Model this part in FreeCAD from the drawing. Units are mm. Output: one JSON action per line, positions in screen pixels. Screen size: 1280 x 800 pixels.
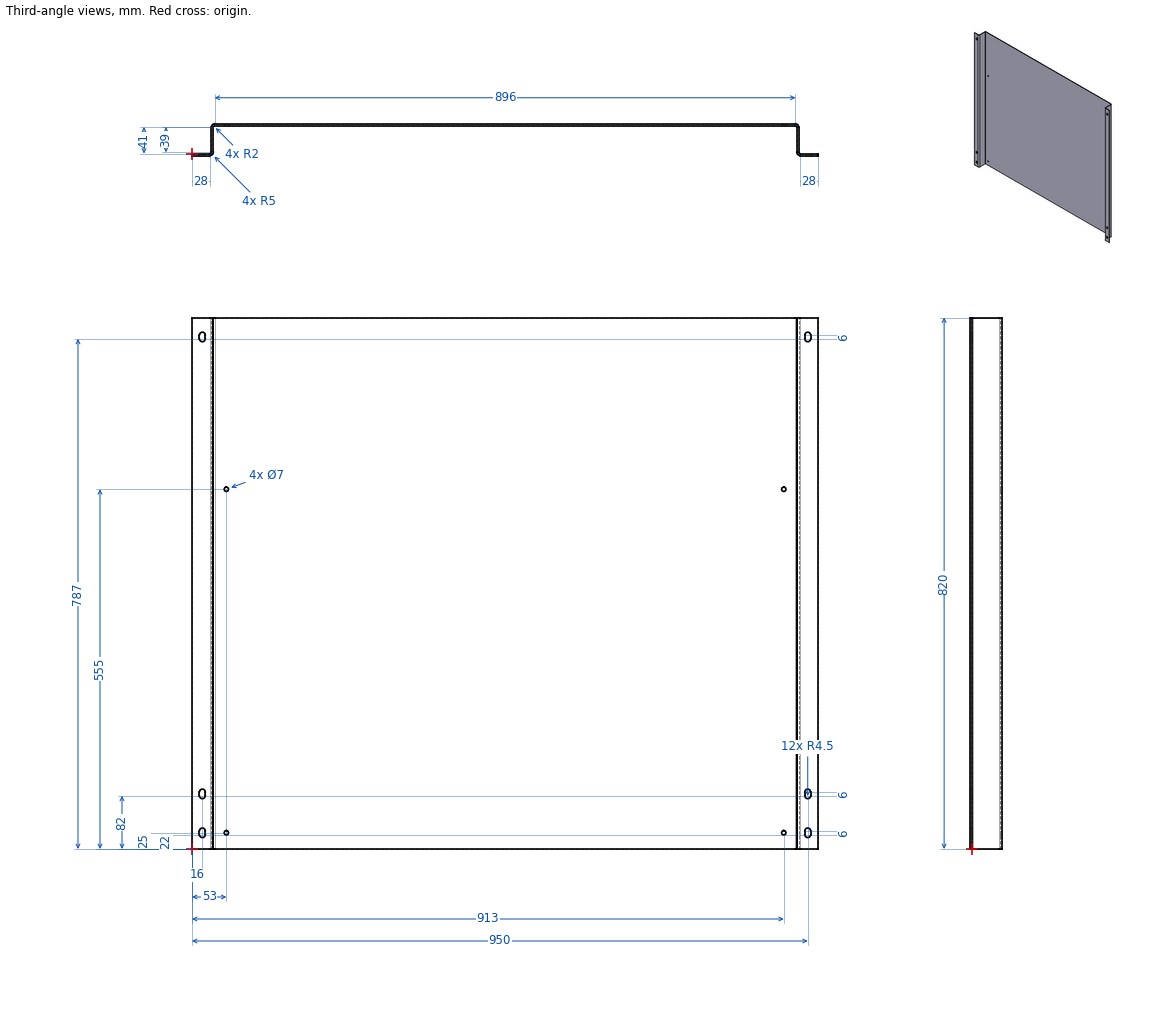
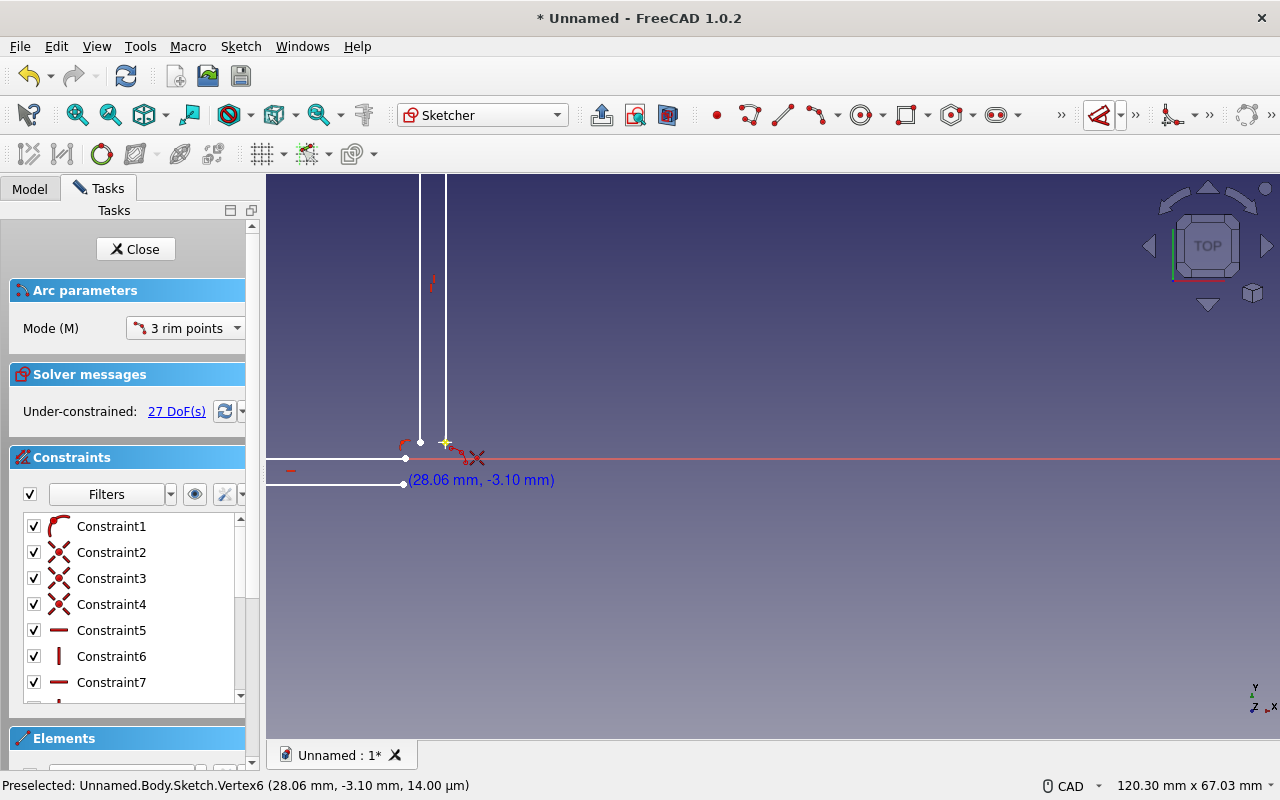
{"action": "left_click", "coordinate": [446, 443]}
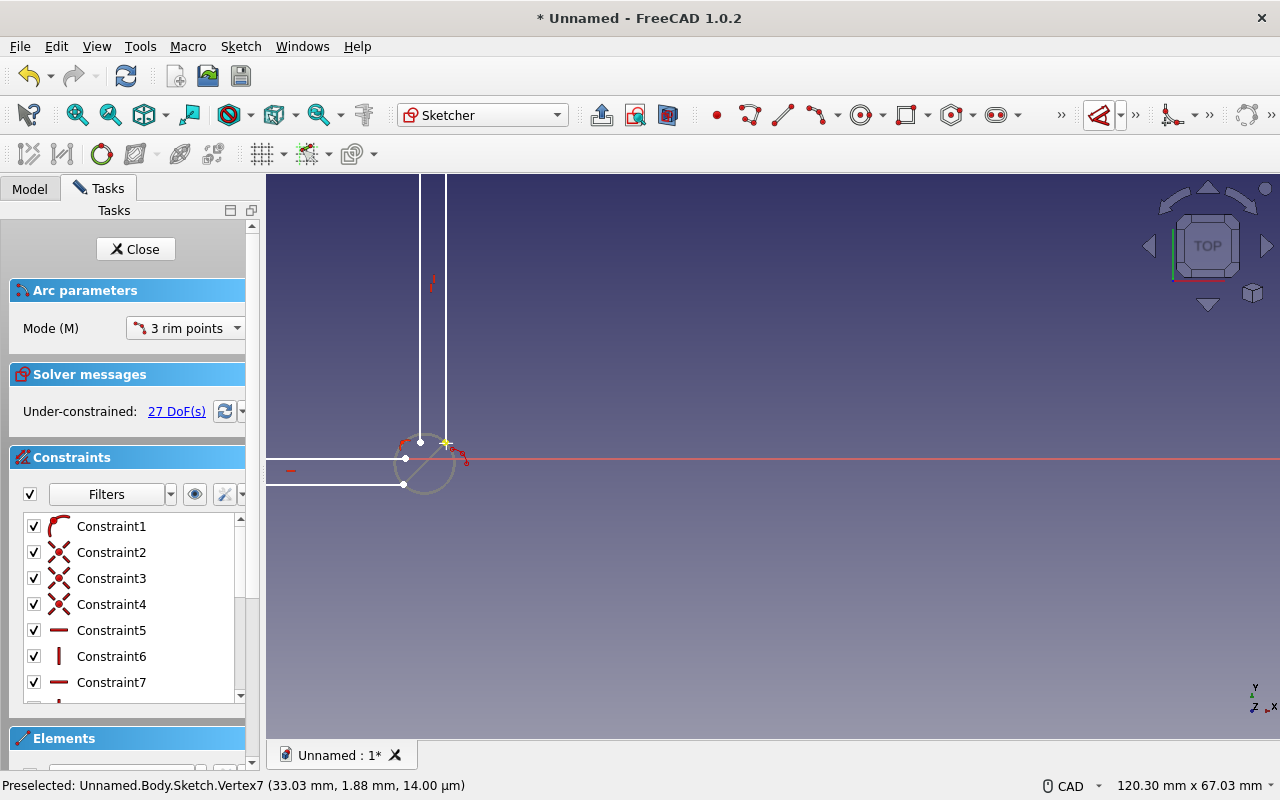
{"action": "scroll", "coordinate": [433, 471], "scroll_direction": "up", "scroll_amount": 2}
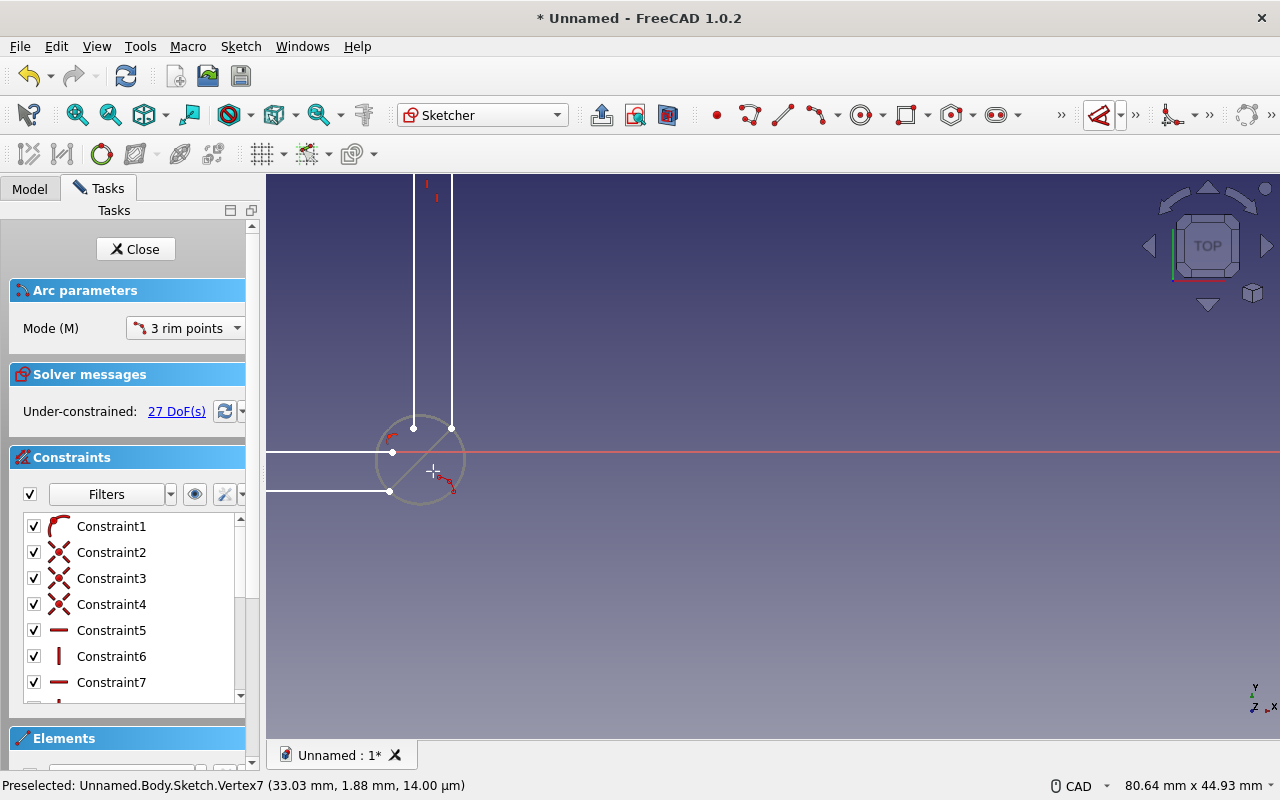
{"action": "left_click", "coordinate": [433, 471]}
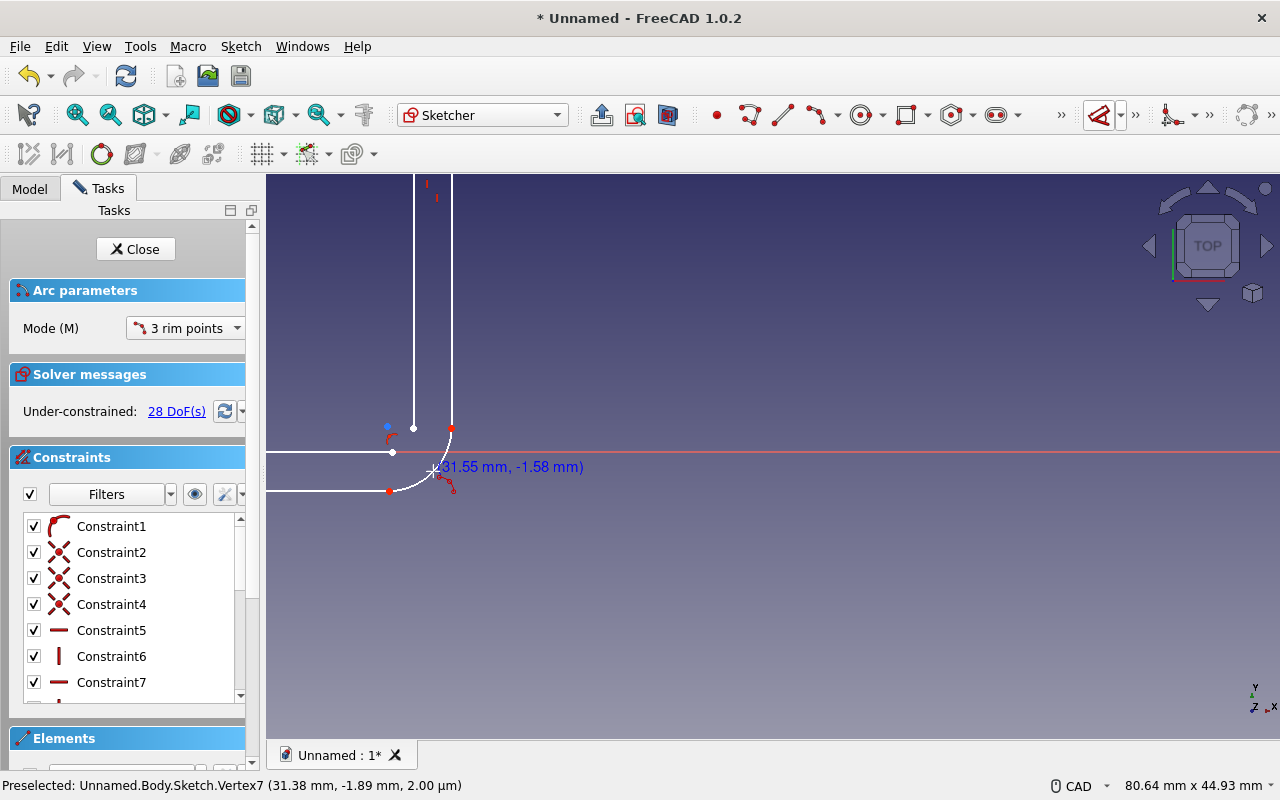
{"action": "scroll", "coordinate": [421, 471], "scroll_direction": "down", "scroll_amount": 15}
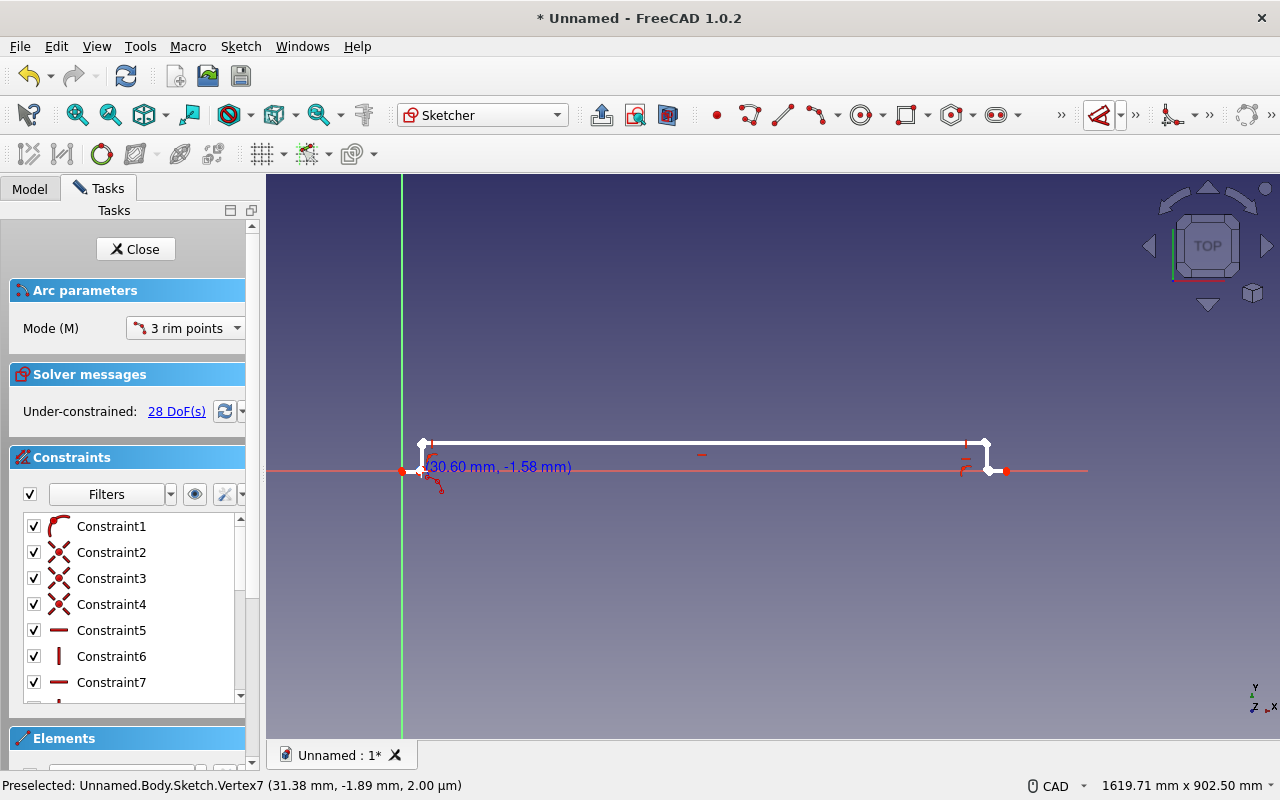
{"action": "scroll", "coordinate": [423, 445], "scroll_direction": "up", "scroll_amount": 11}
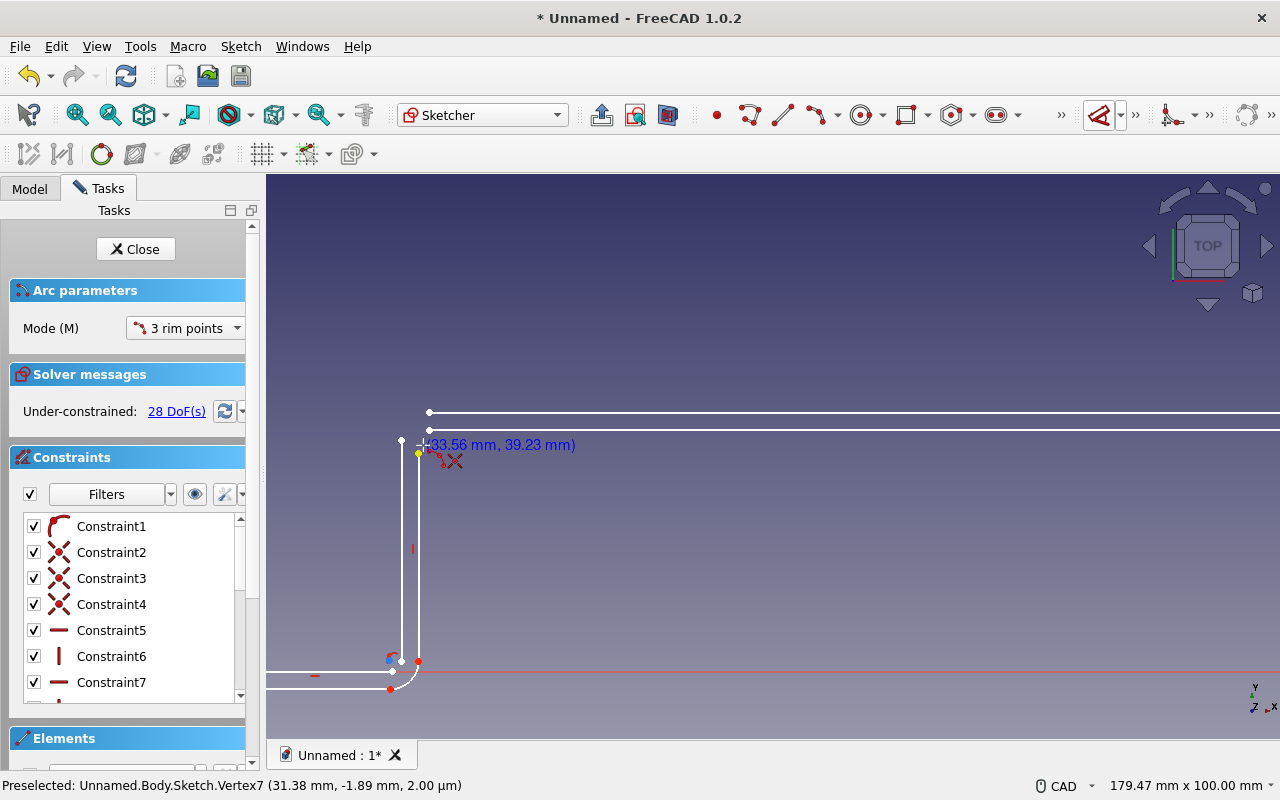
{"action": "left_click", "coordinate": [423, 444]}
{"action": "left_click", "coordinate": [430, 430]}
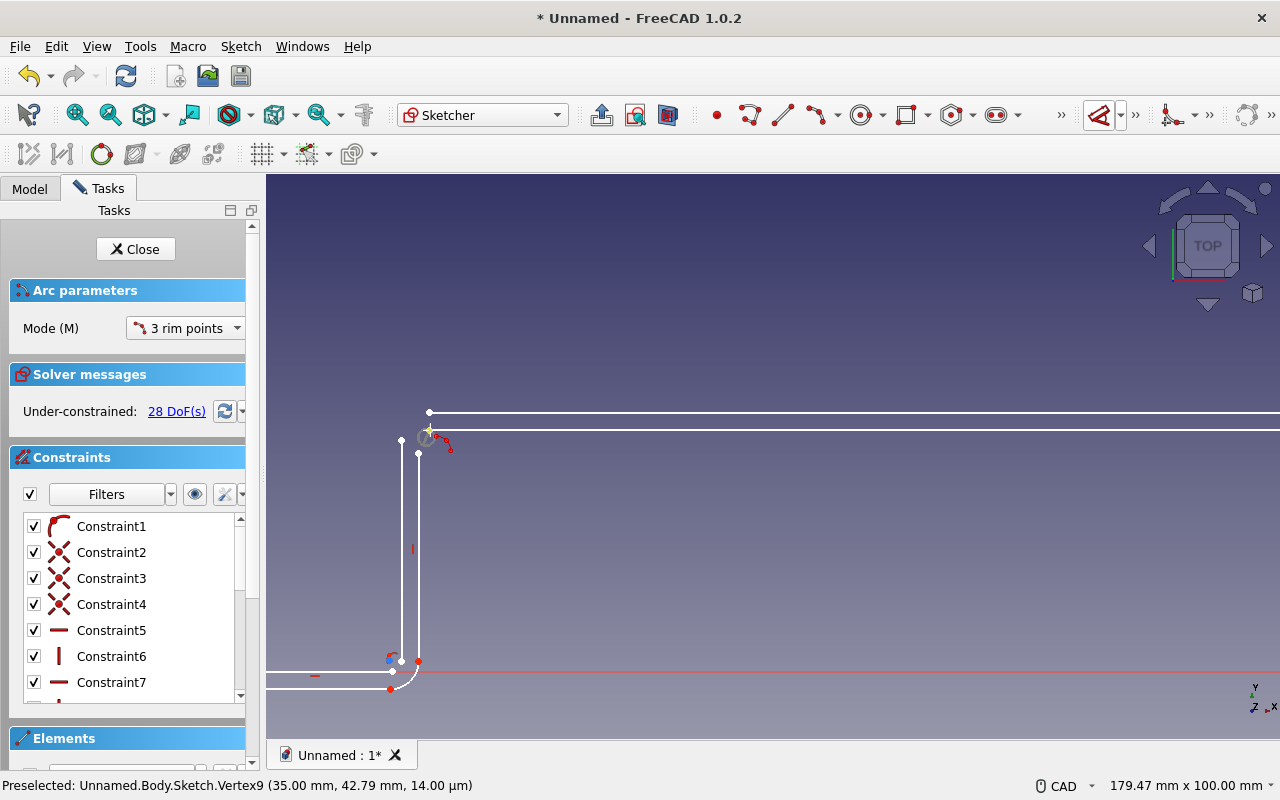
{"action": "scroll", "coordinate": [422, 432], "scroll_direction": "up", "scroll_amount": 8}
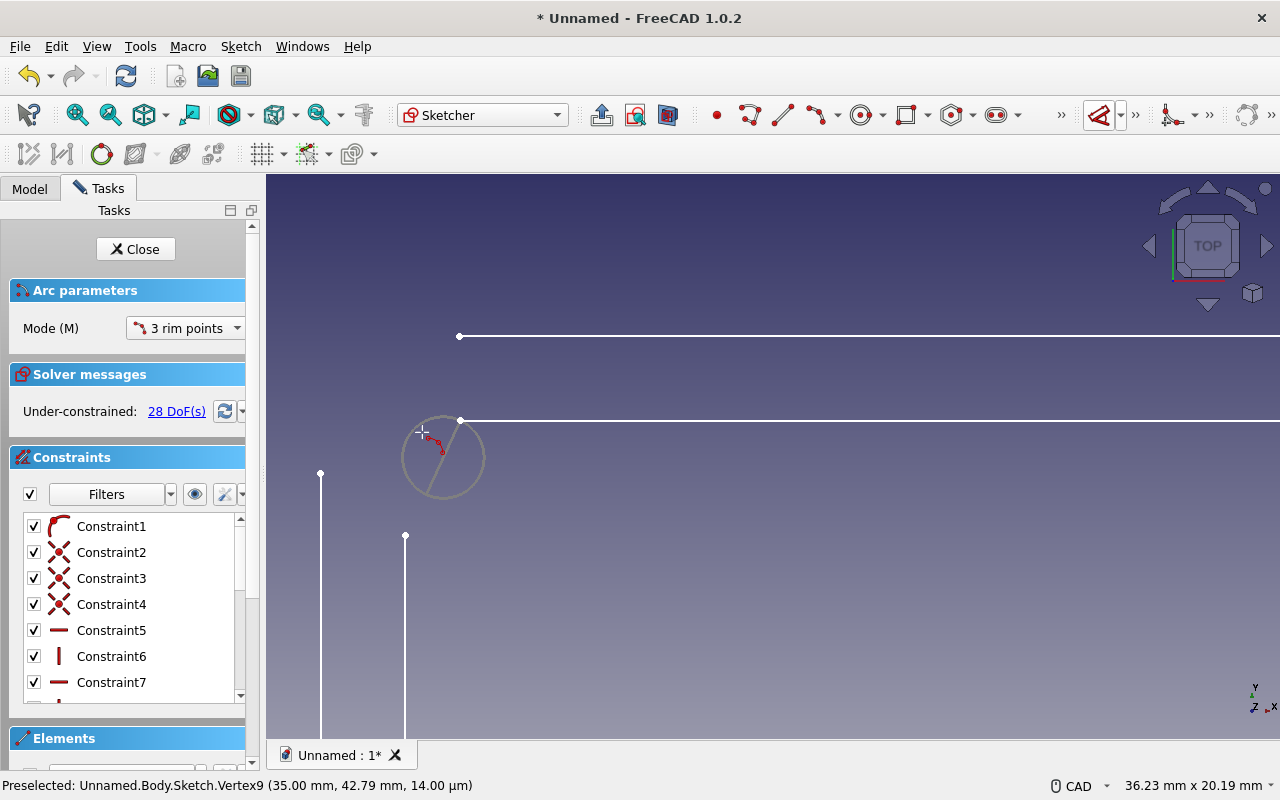
{"action": "left_click", "coordinate": [421, 431]}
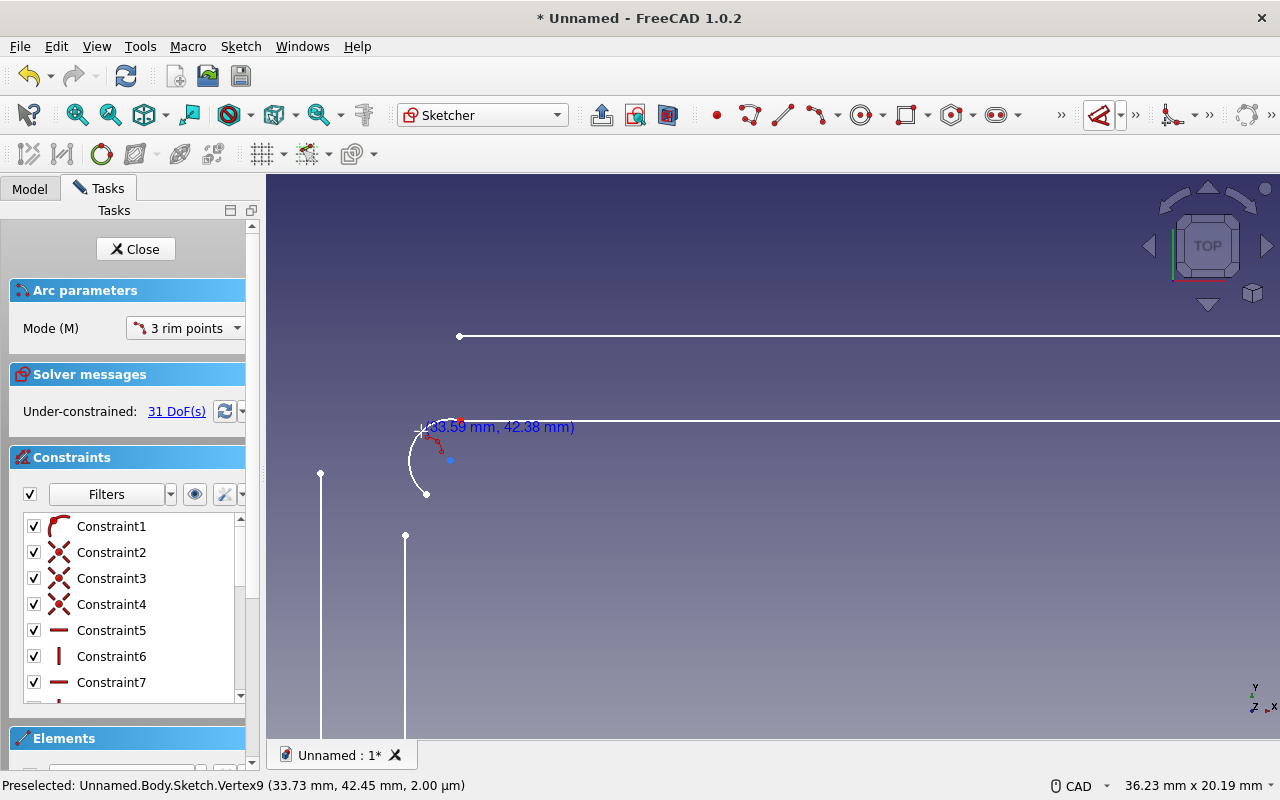
{"action": "scroll", "coordinate": [359, 441], "scroll_direction": "down", "scroll_amount": 18}